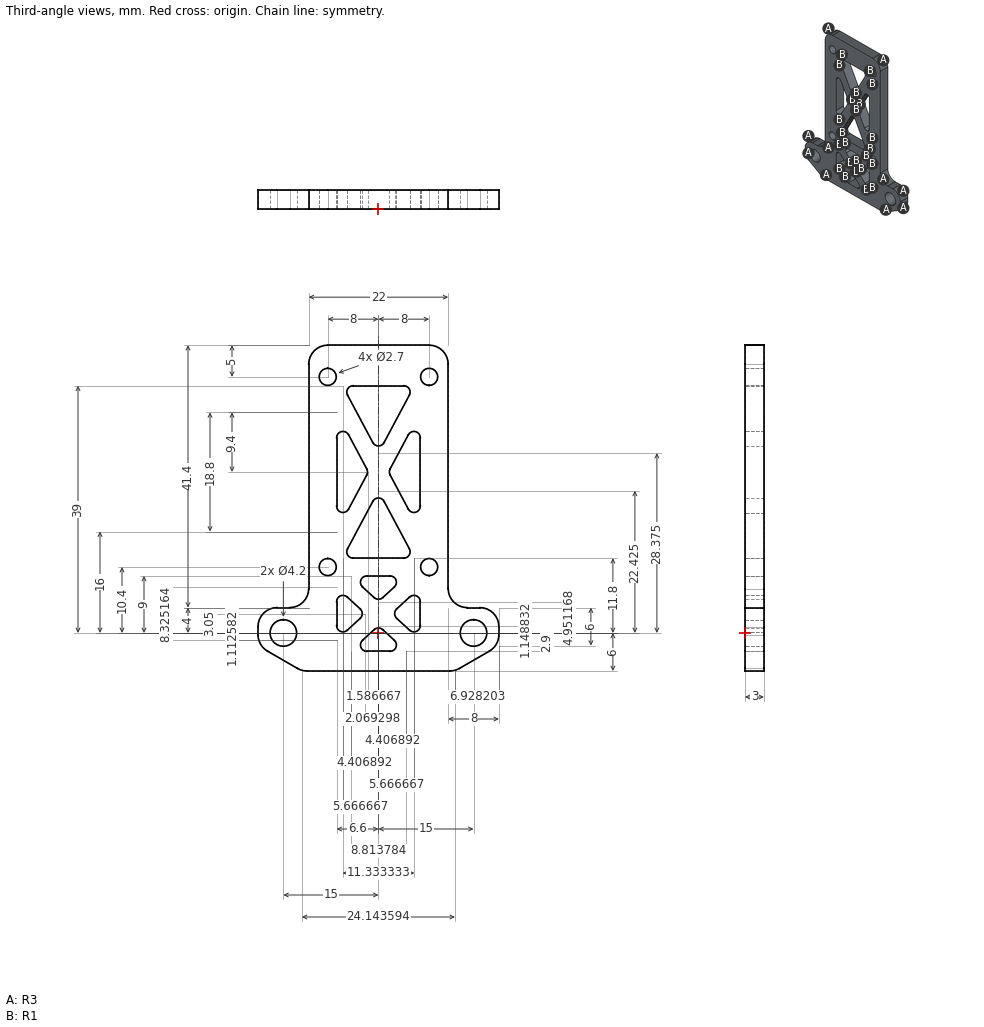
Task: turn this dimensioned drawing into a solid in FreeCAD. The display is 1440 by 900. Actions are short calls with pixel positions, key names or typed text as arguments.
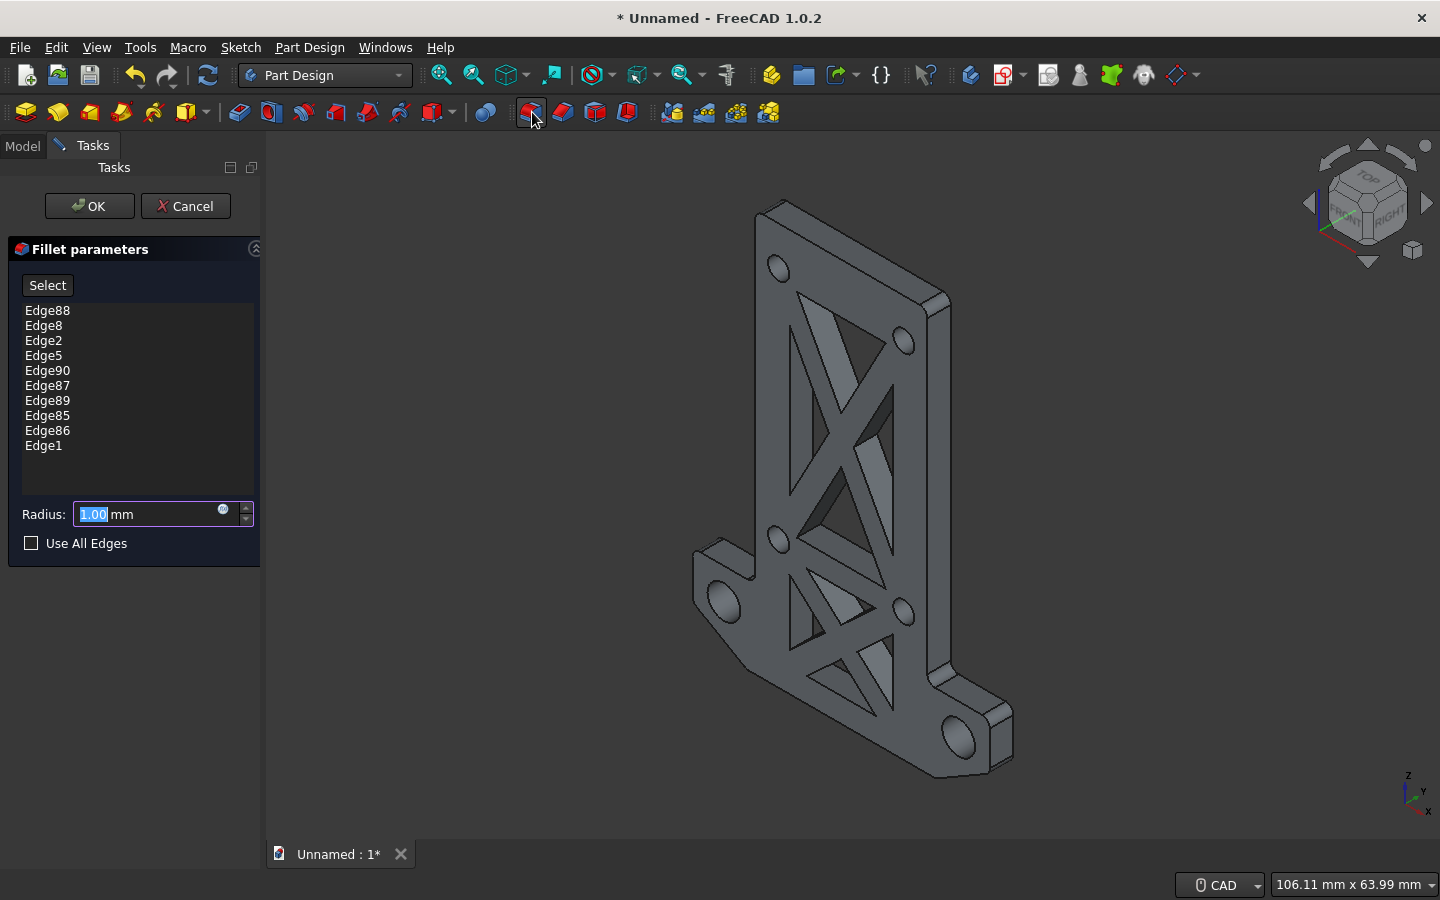
text(3)
key(Tab)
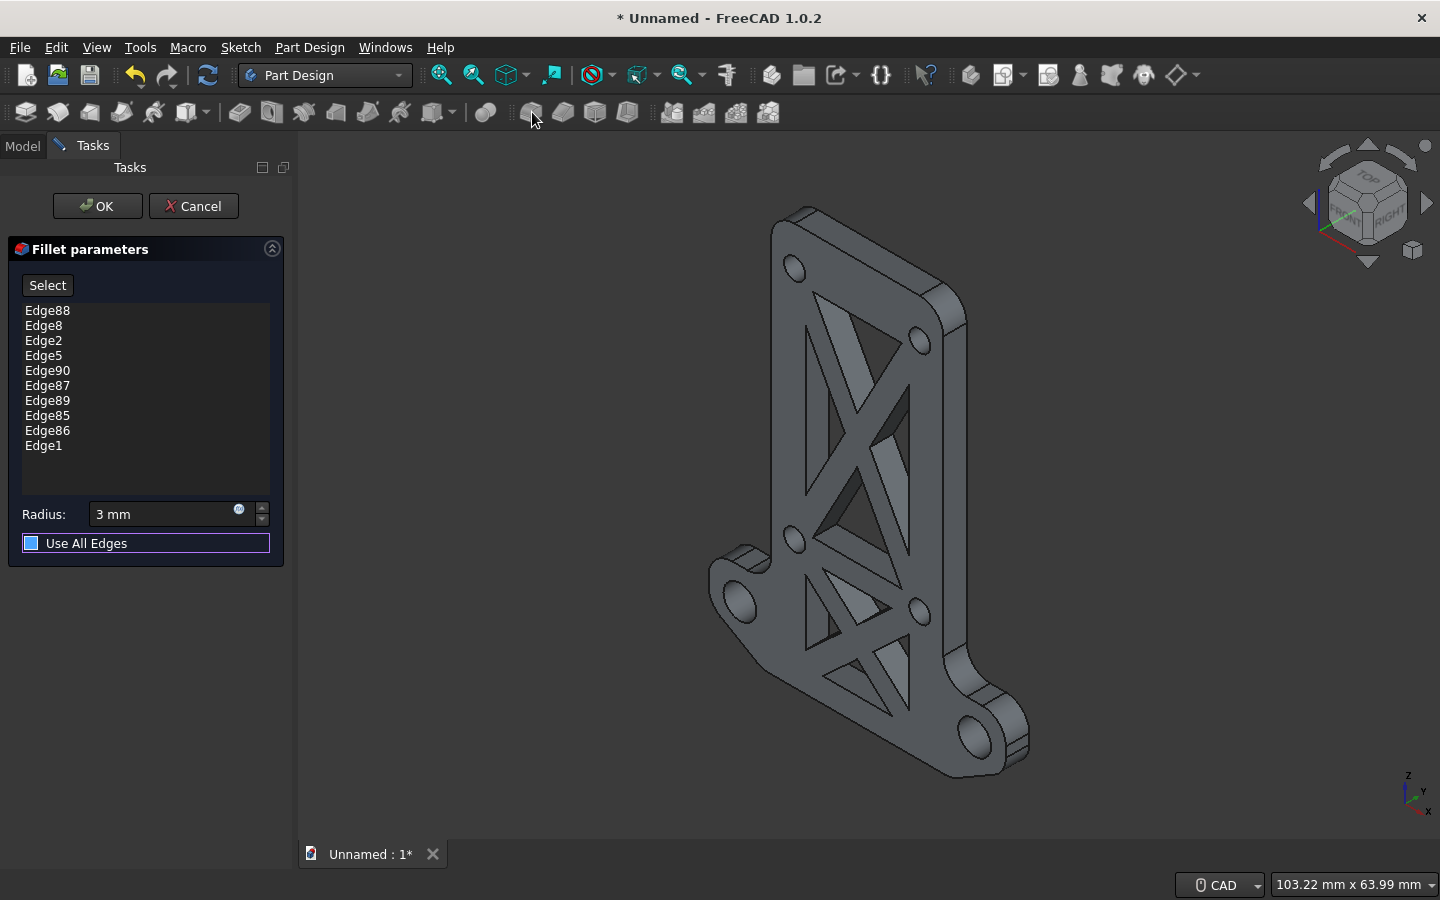
click(98, 206)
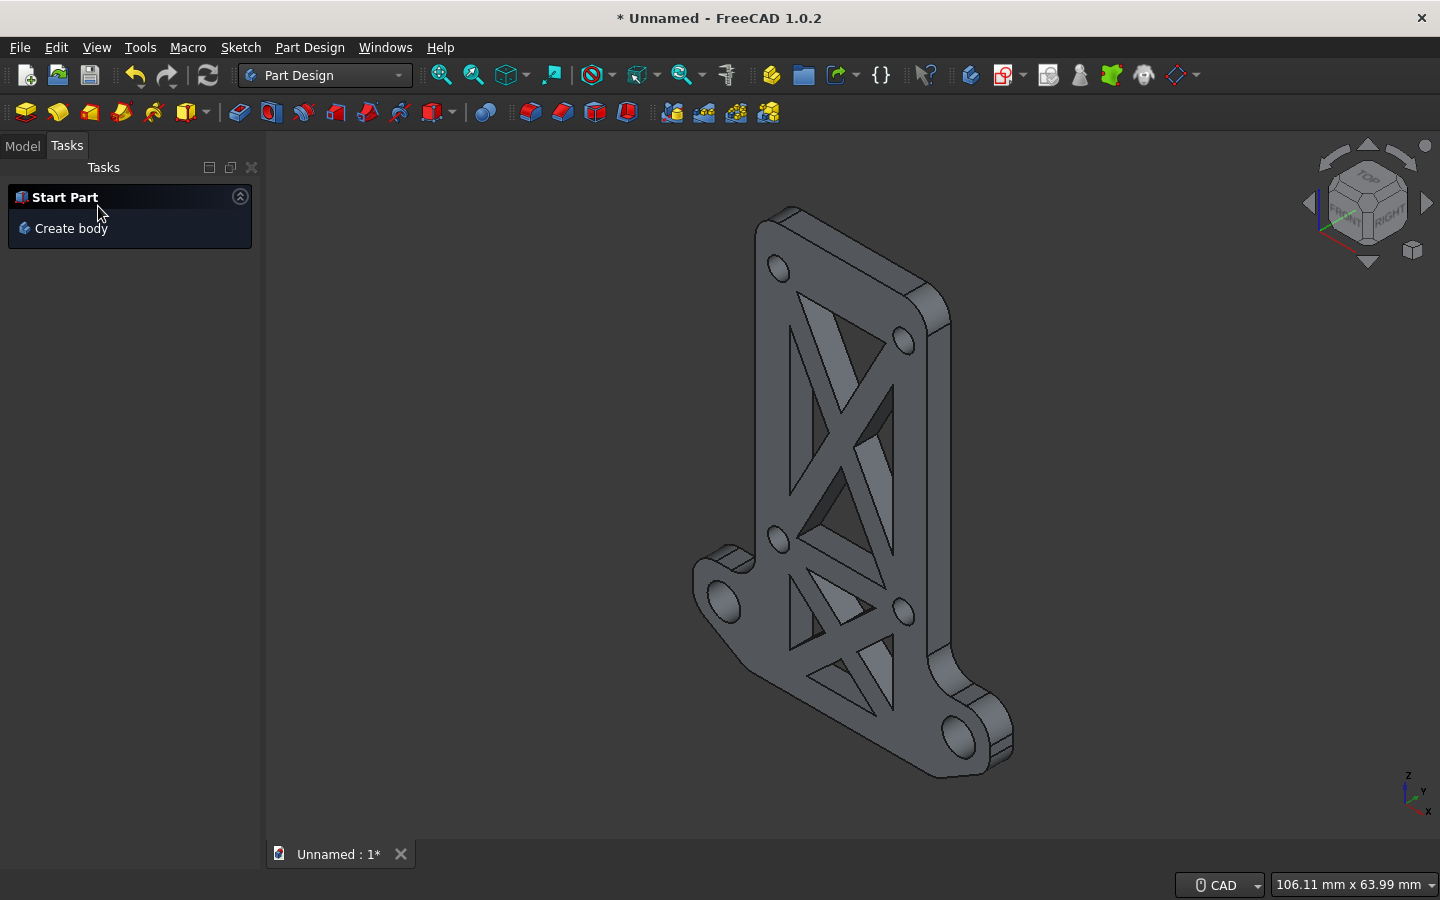
key(2)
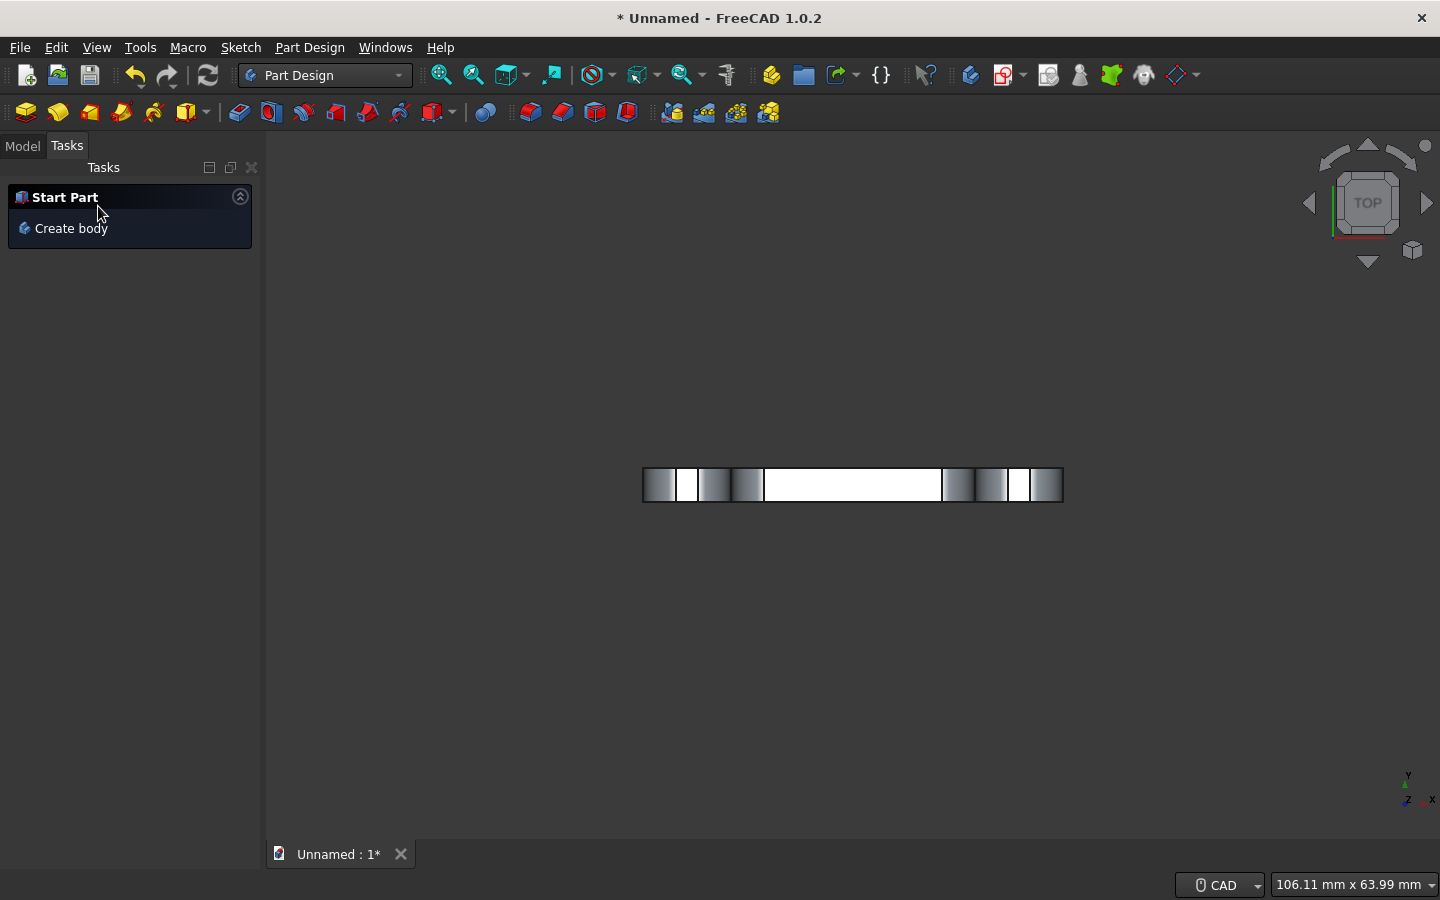
key(v)
key(f)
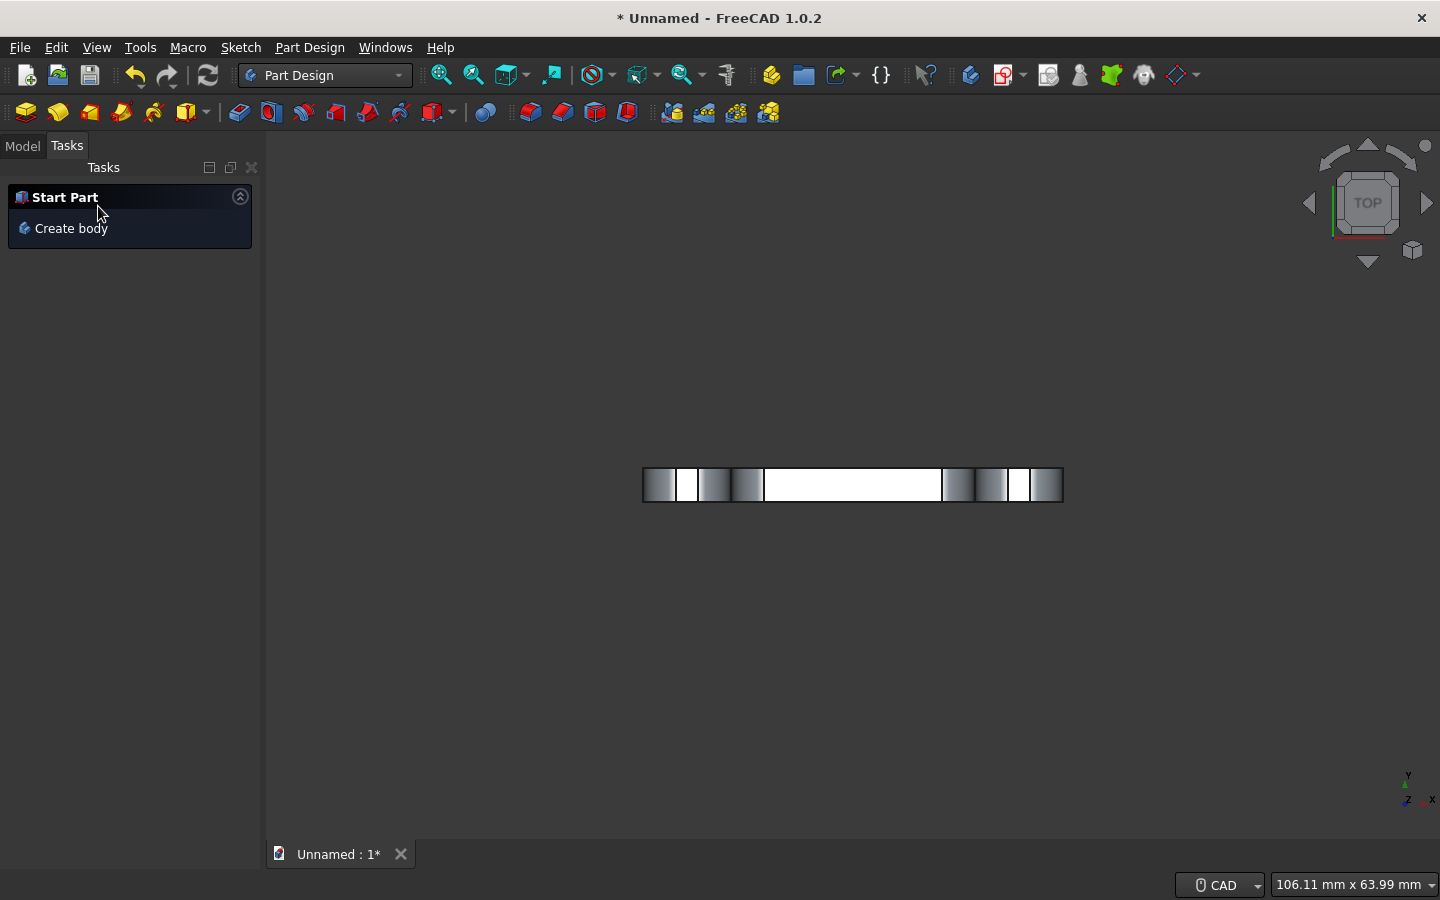
key(0)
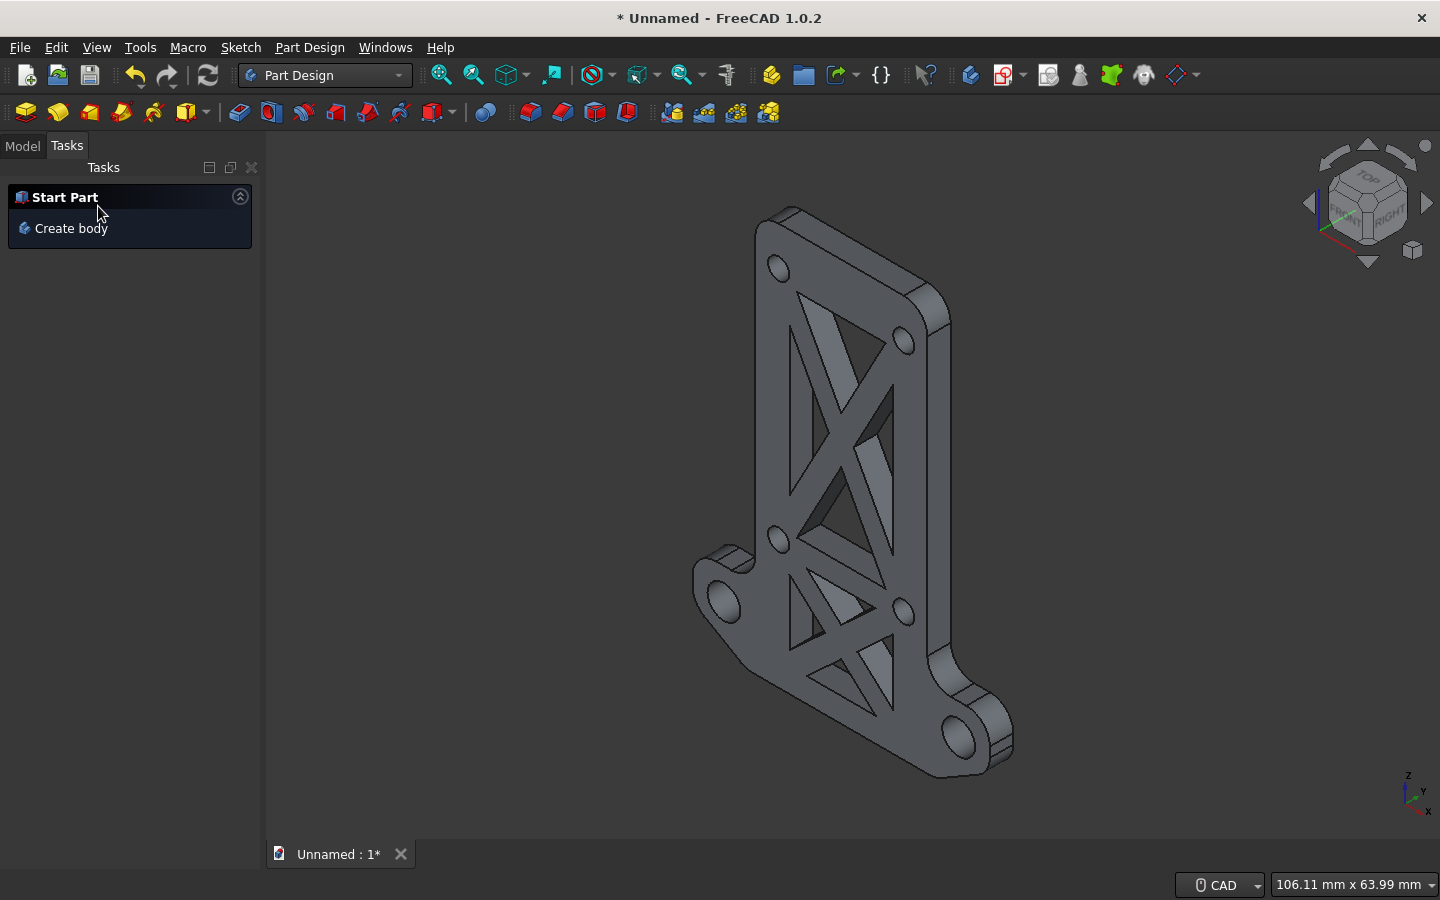
key(1)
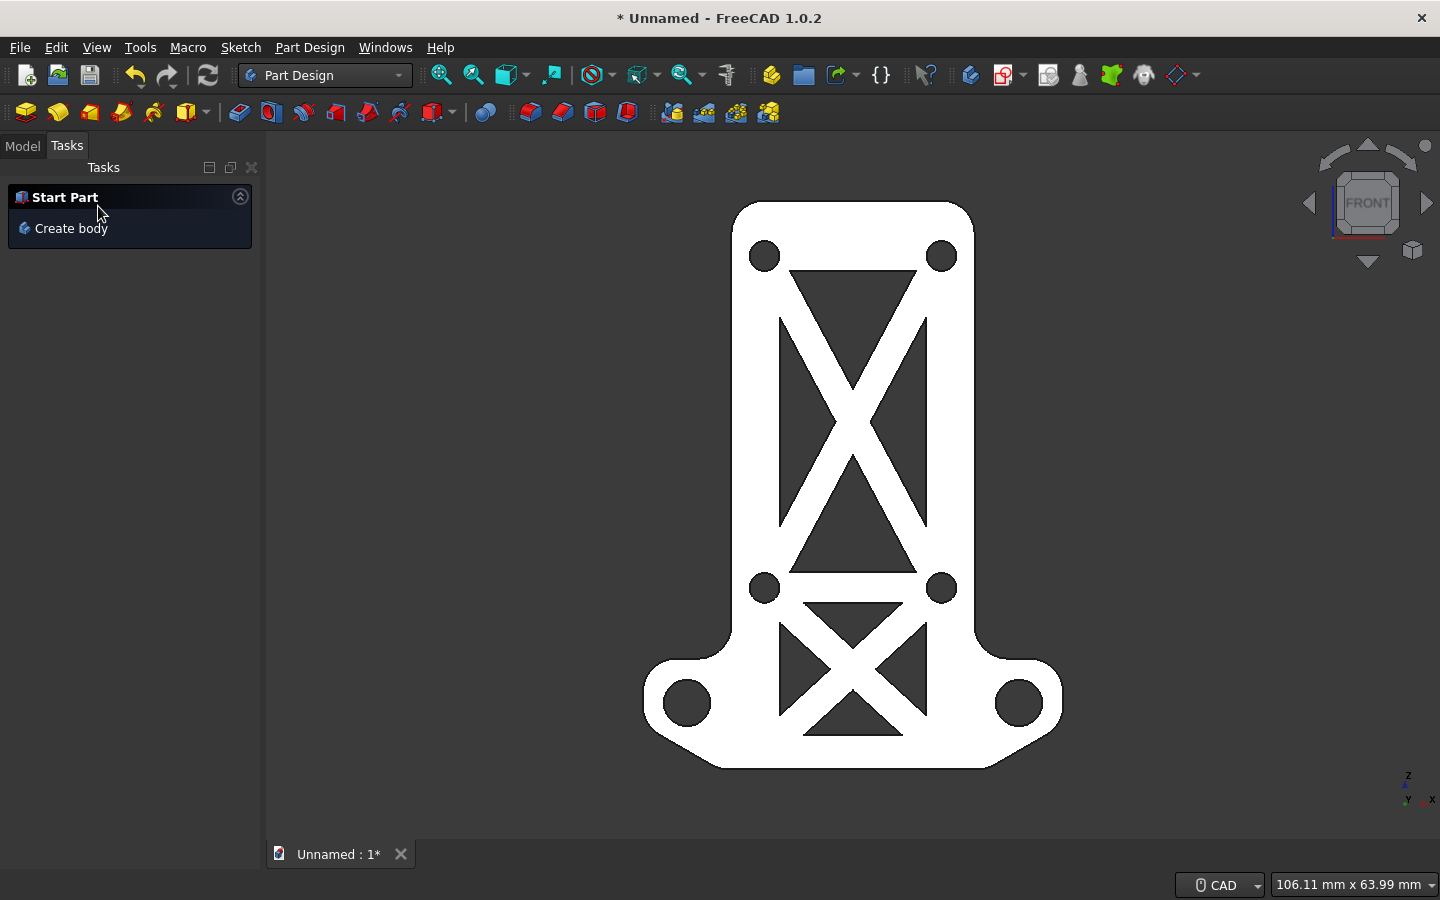
key(3)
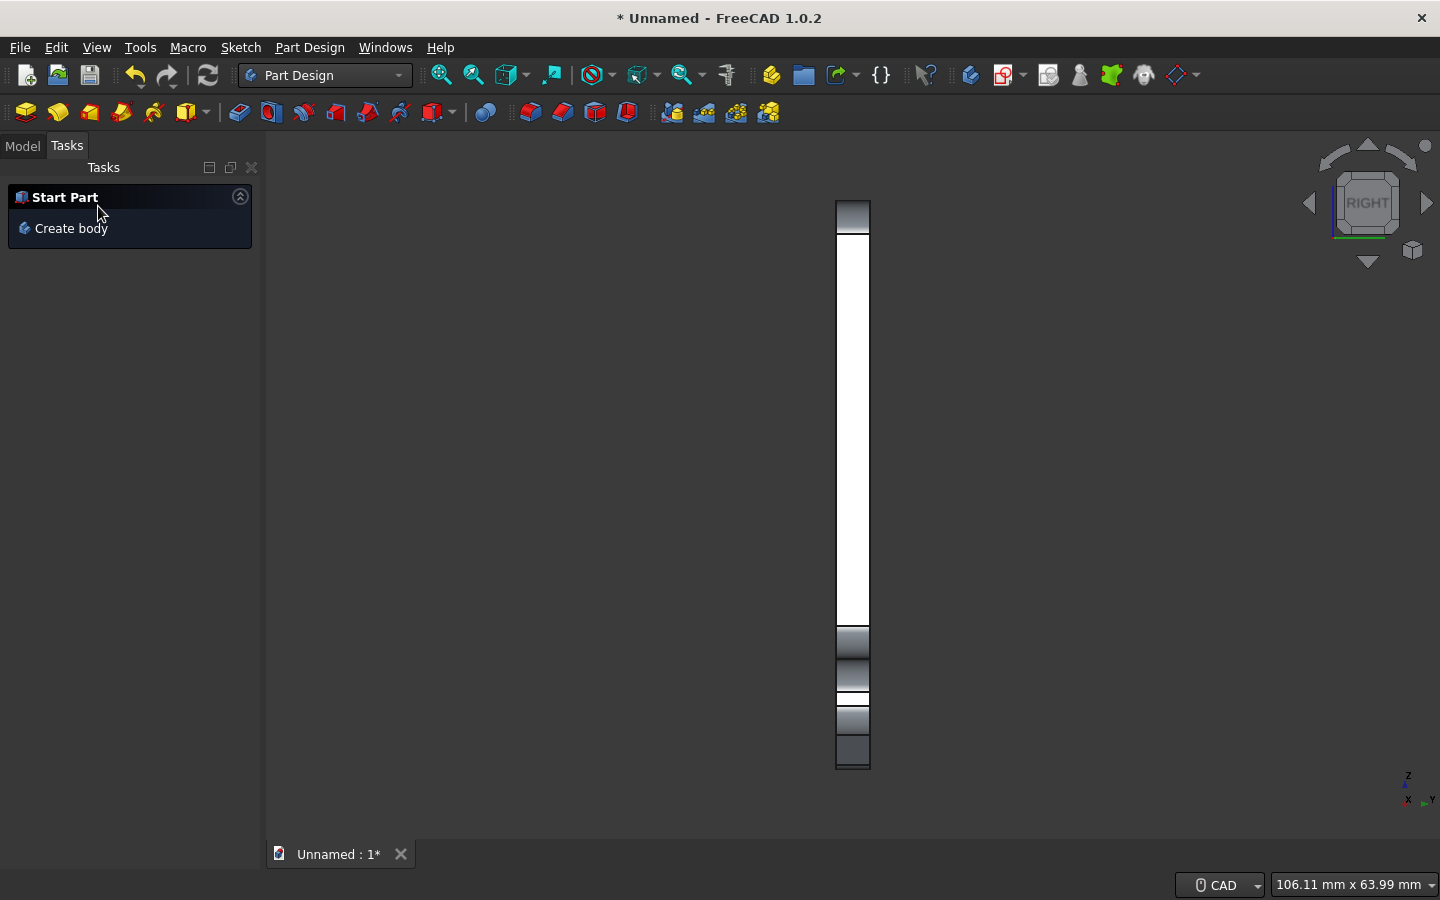
key(5)